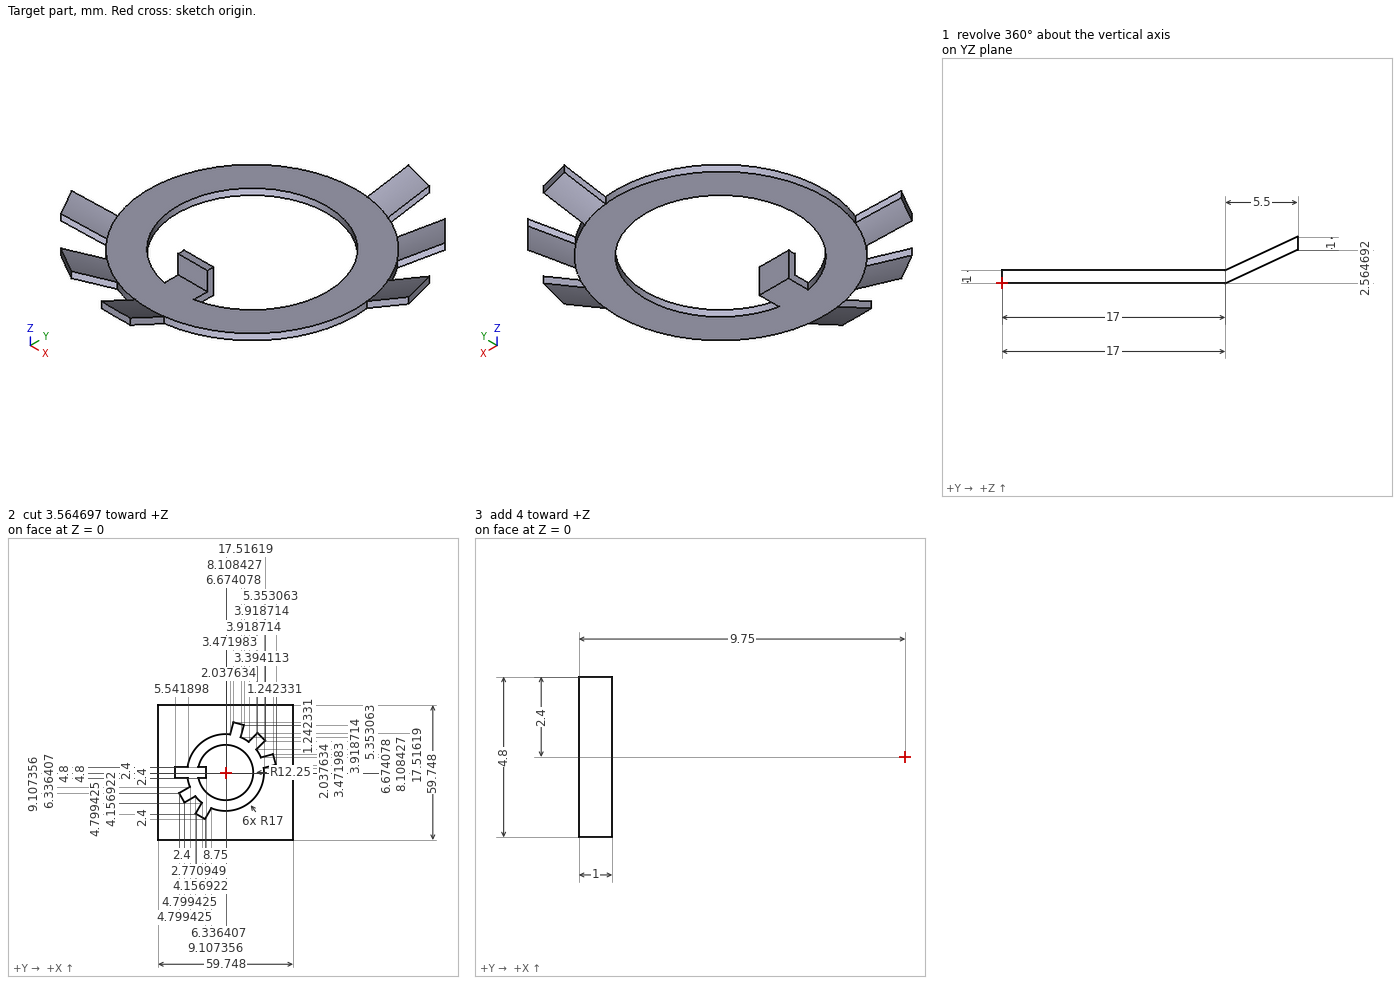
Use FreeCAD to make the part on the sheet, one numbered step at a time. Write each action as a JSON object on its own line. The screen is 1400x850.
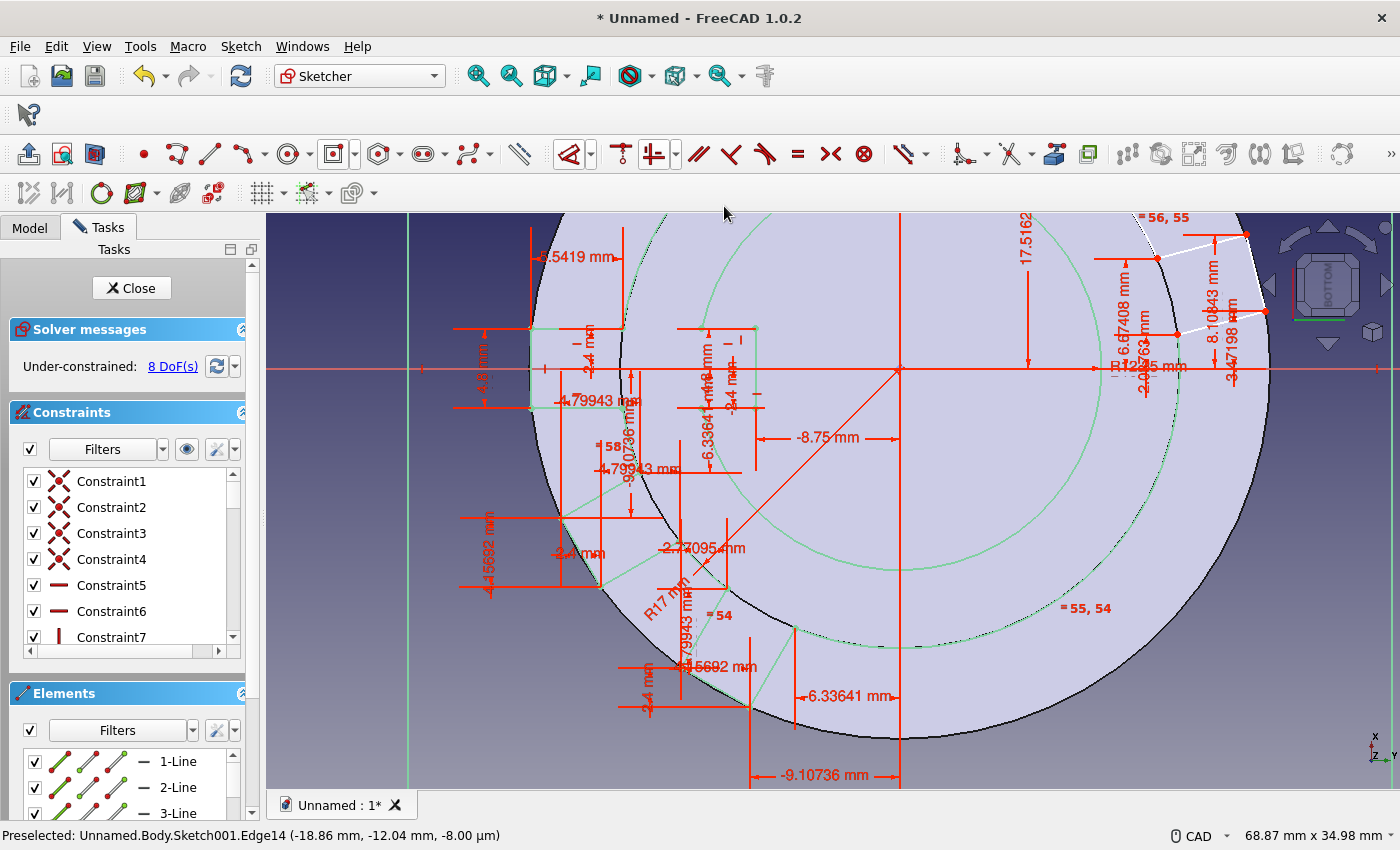
{"action": "left_click", "coordinate": [1204, 328]}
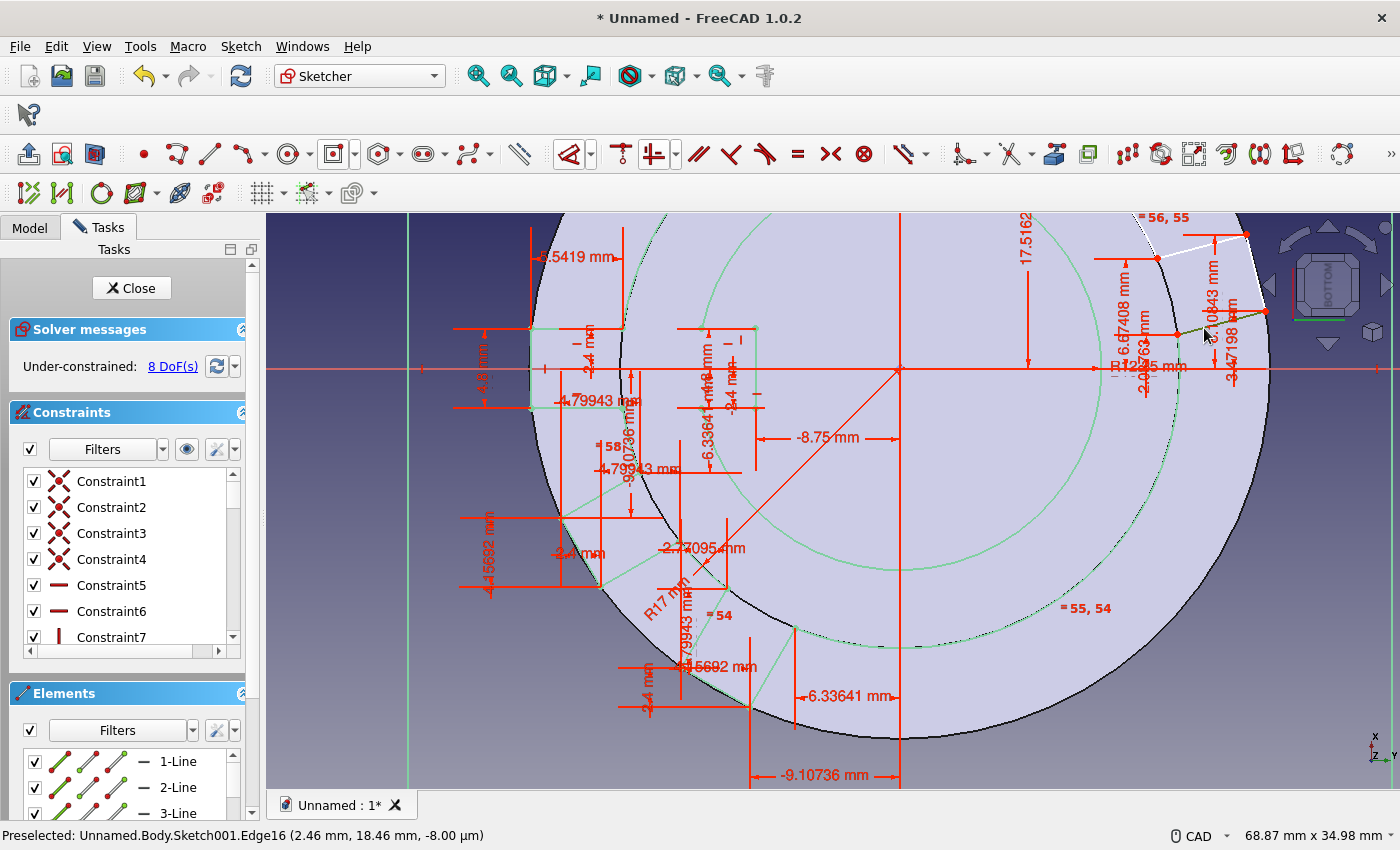
{"action": "left_click", "coordinate": [590, 154]}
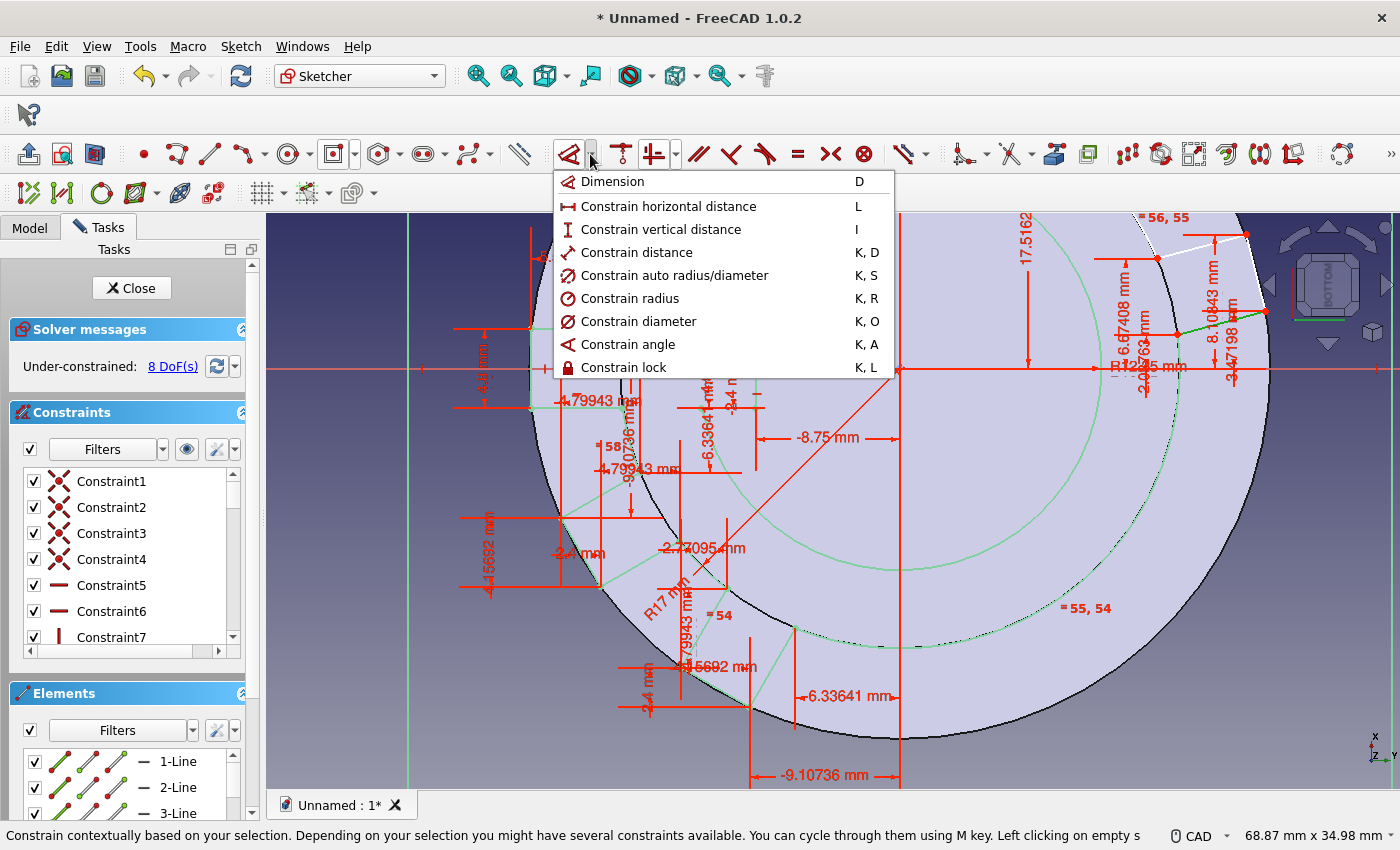
{"action": "left_click", "coordinate": [724, 206]}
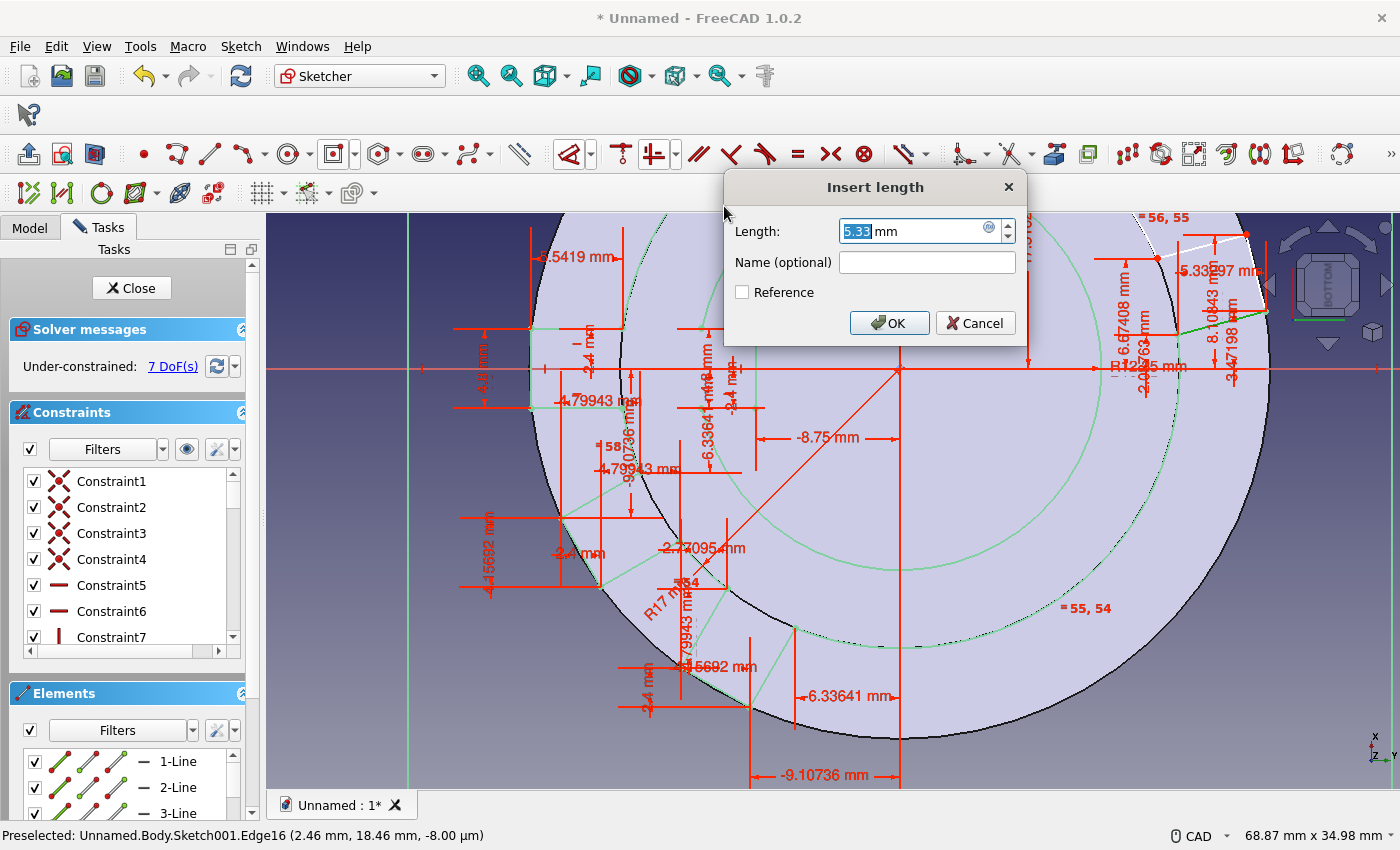
{"action": "type", "text": "5.353063"}
{"action": "key", "text": "Return"}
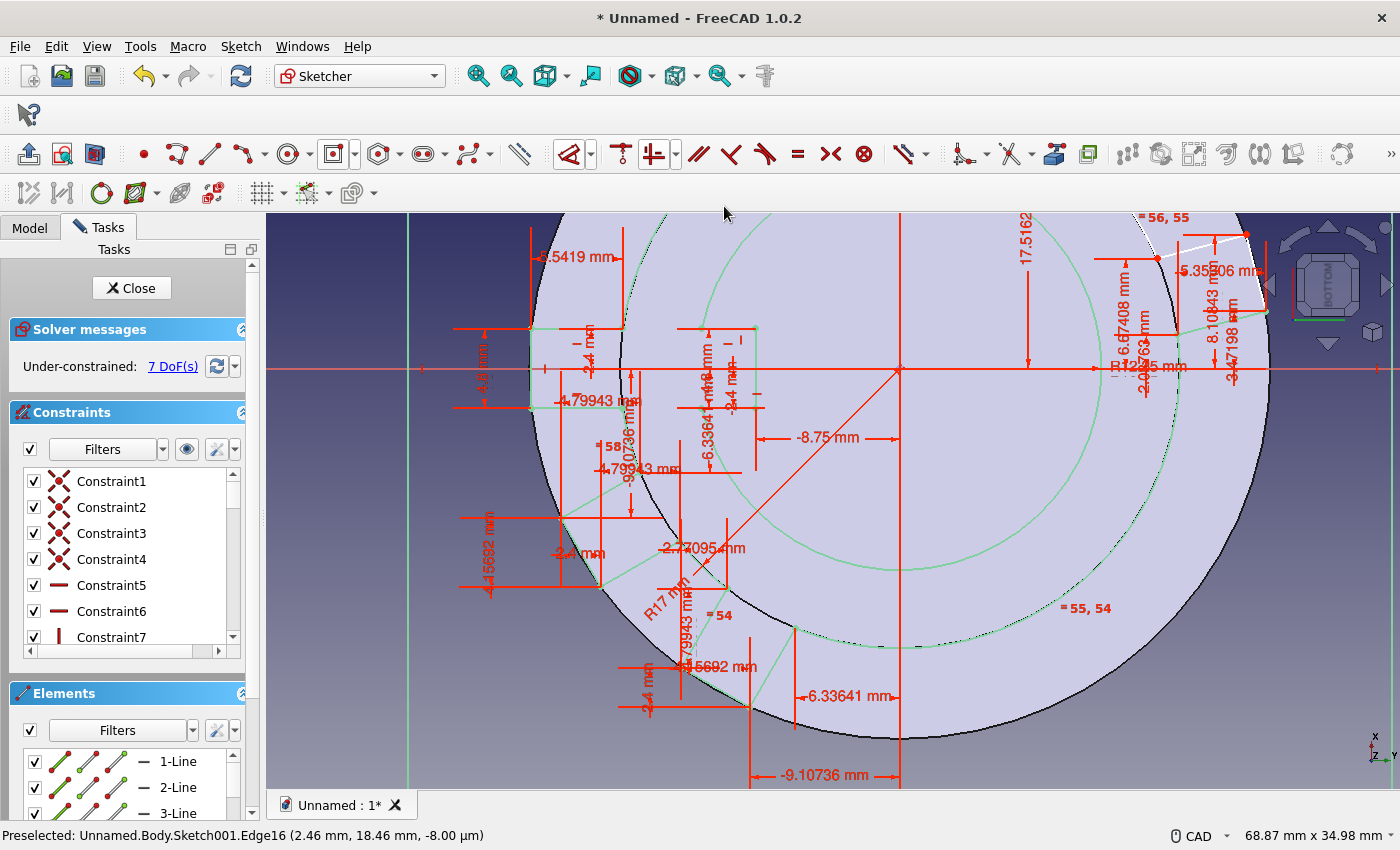
{"action": "scroll", "coordinate": [686, 578], "scroll_direction": "down", "scroll_amount": 5}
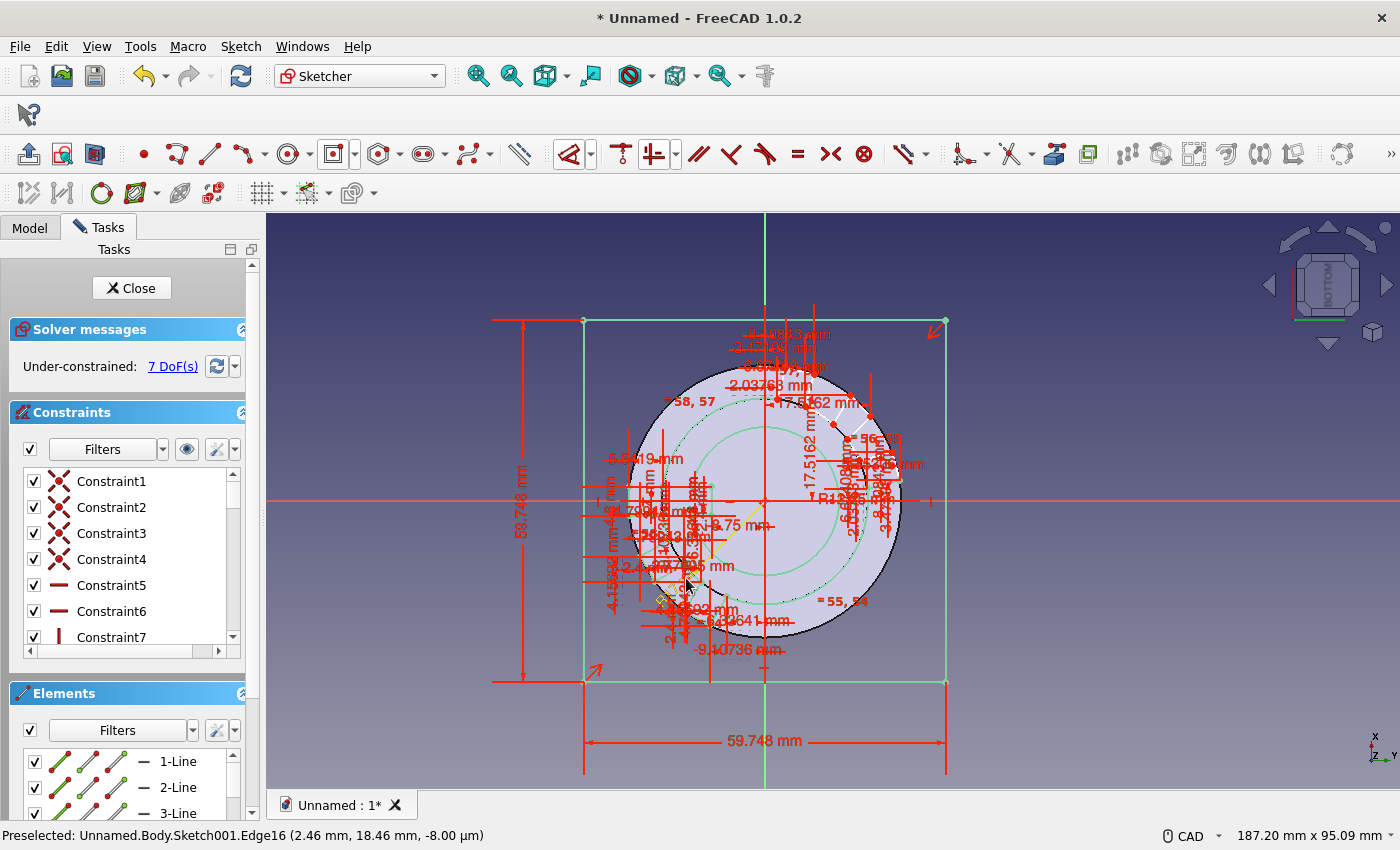
{"action": "scroll", "coordinate": [897, 472], "scroll_direction": "up", "scroll_amount": 9}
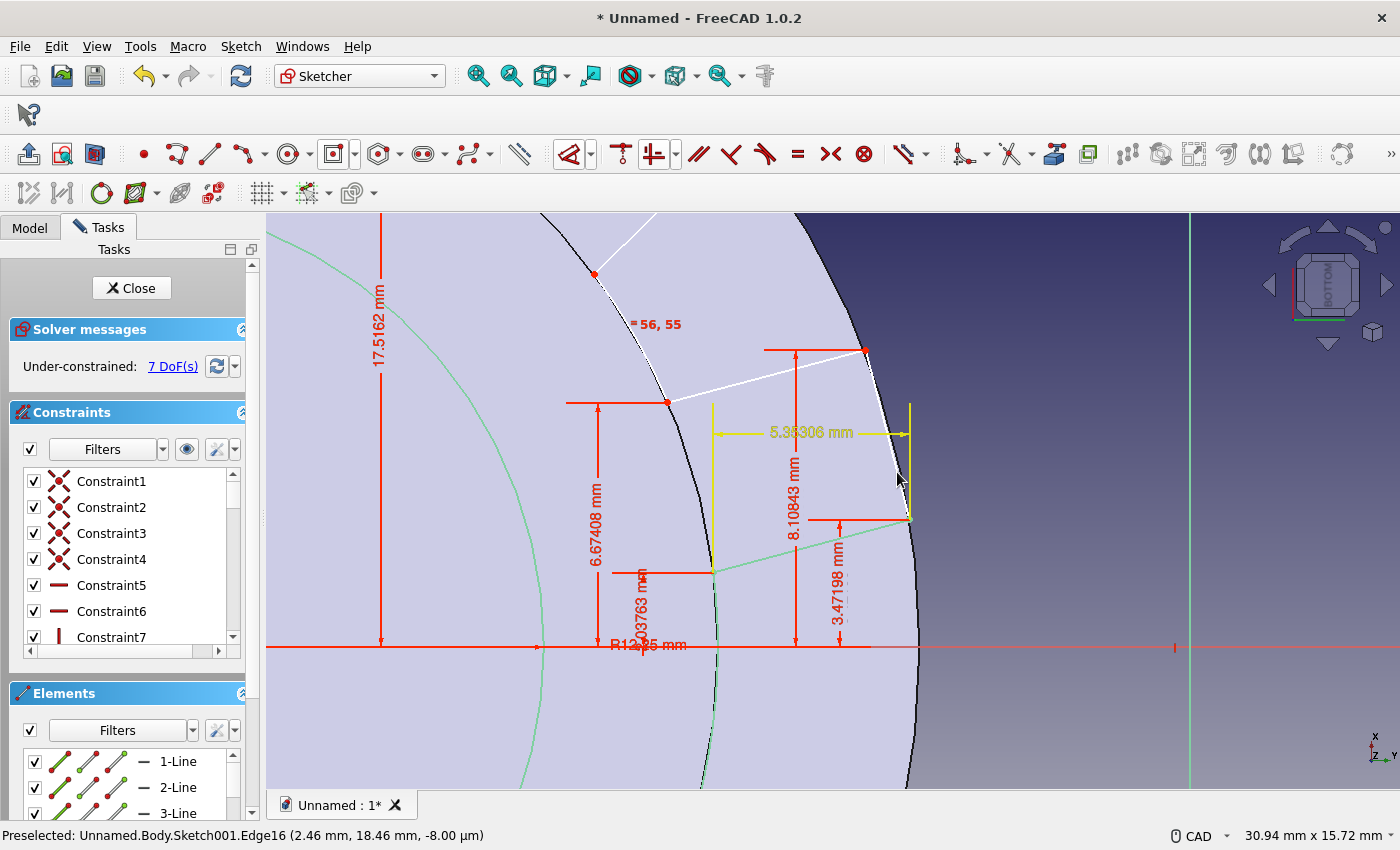
{"action": "left_click", "coordinate": [896, 469]}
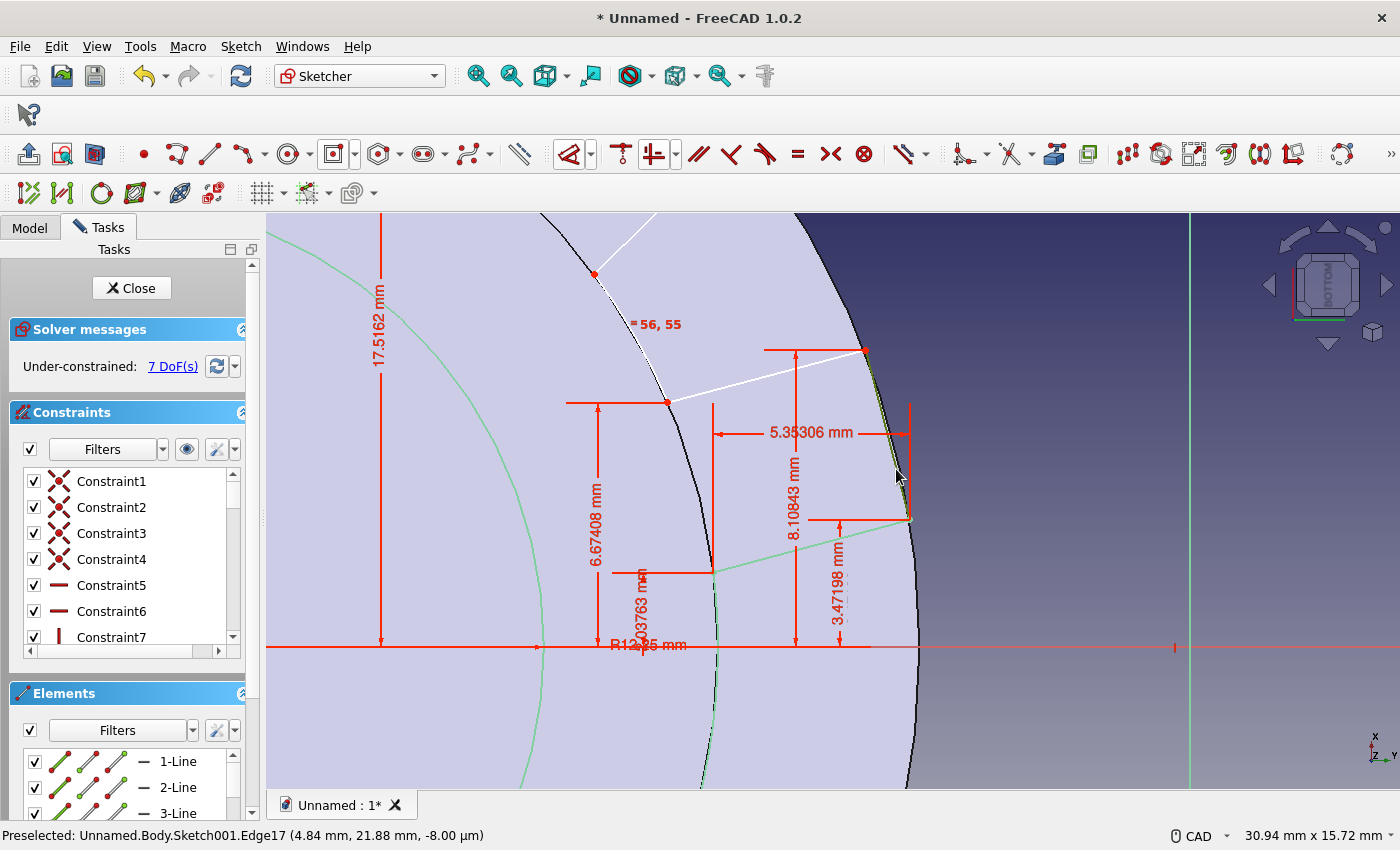
{"action": "key", "text": "l"}